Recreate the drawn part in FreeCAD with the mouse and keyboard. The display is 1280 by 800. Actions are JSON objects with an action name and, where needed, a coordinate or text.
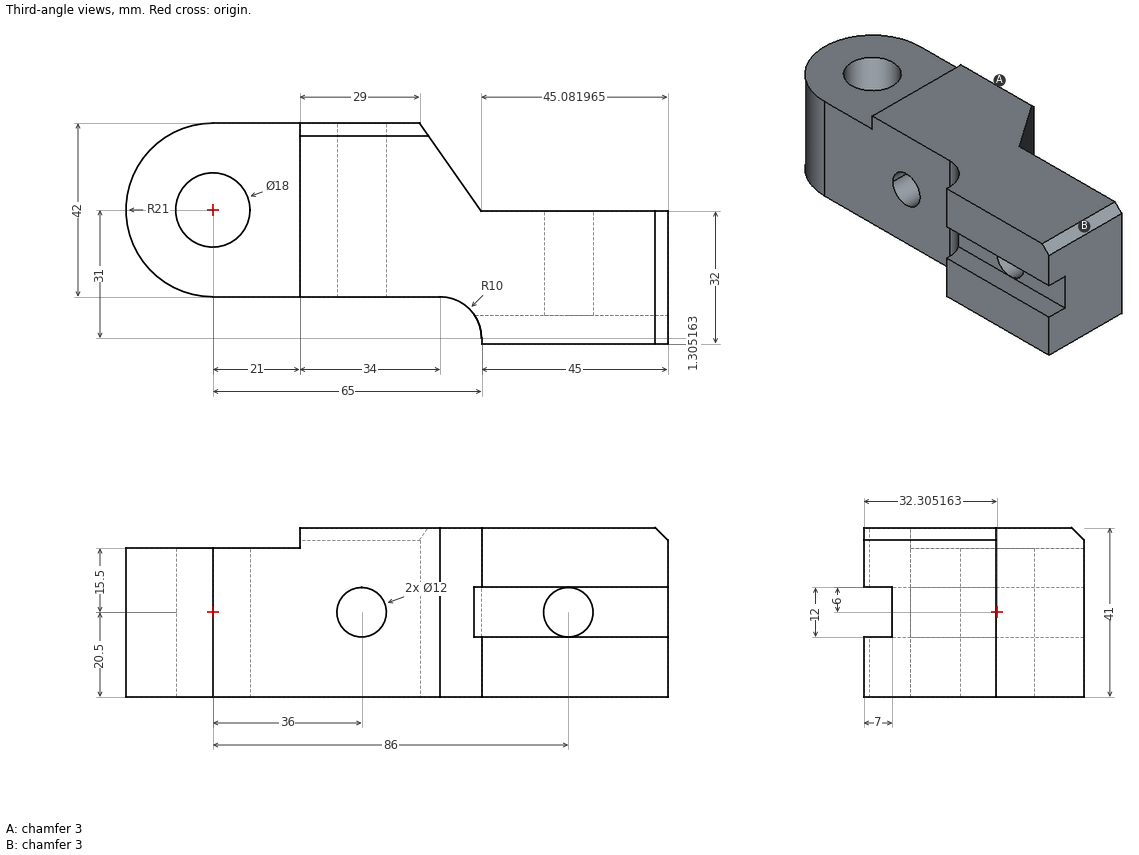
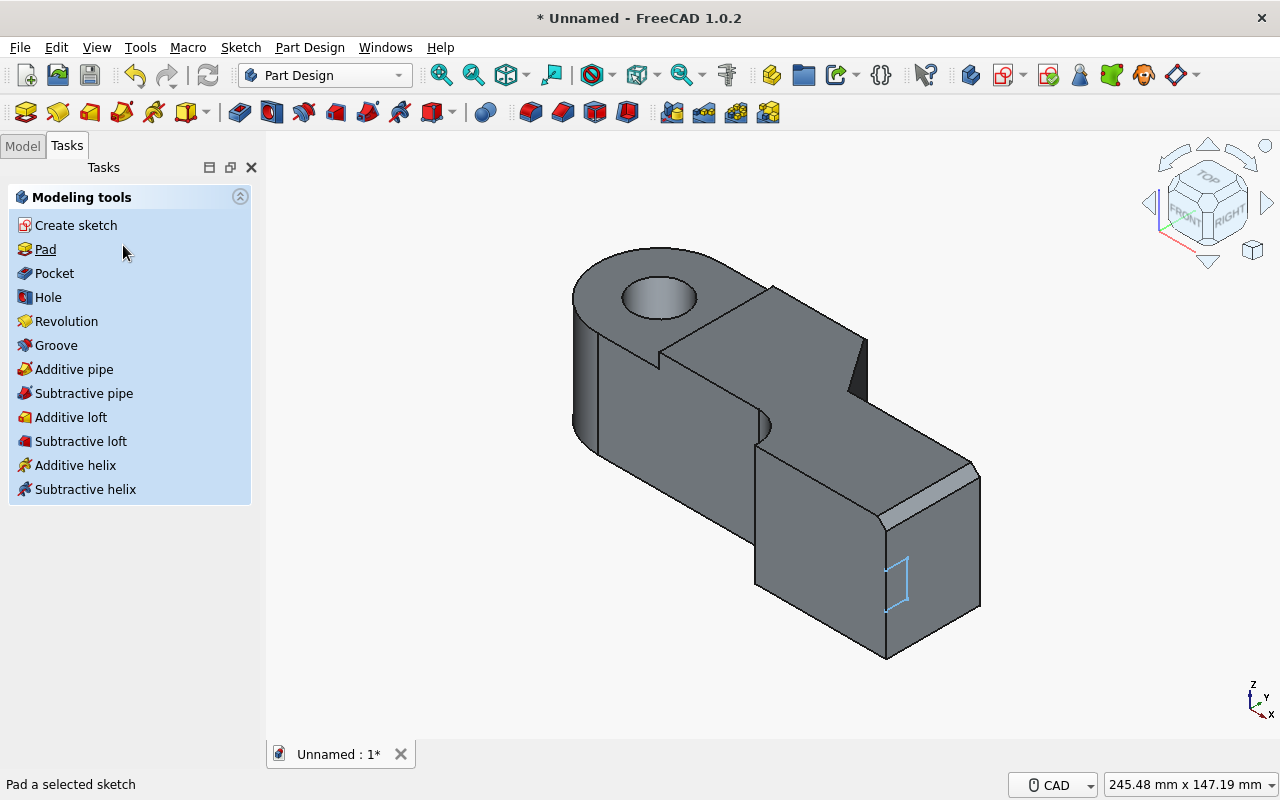
{"action": "left_click", "coordinate": [240, 112]}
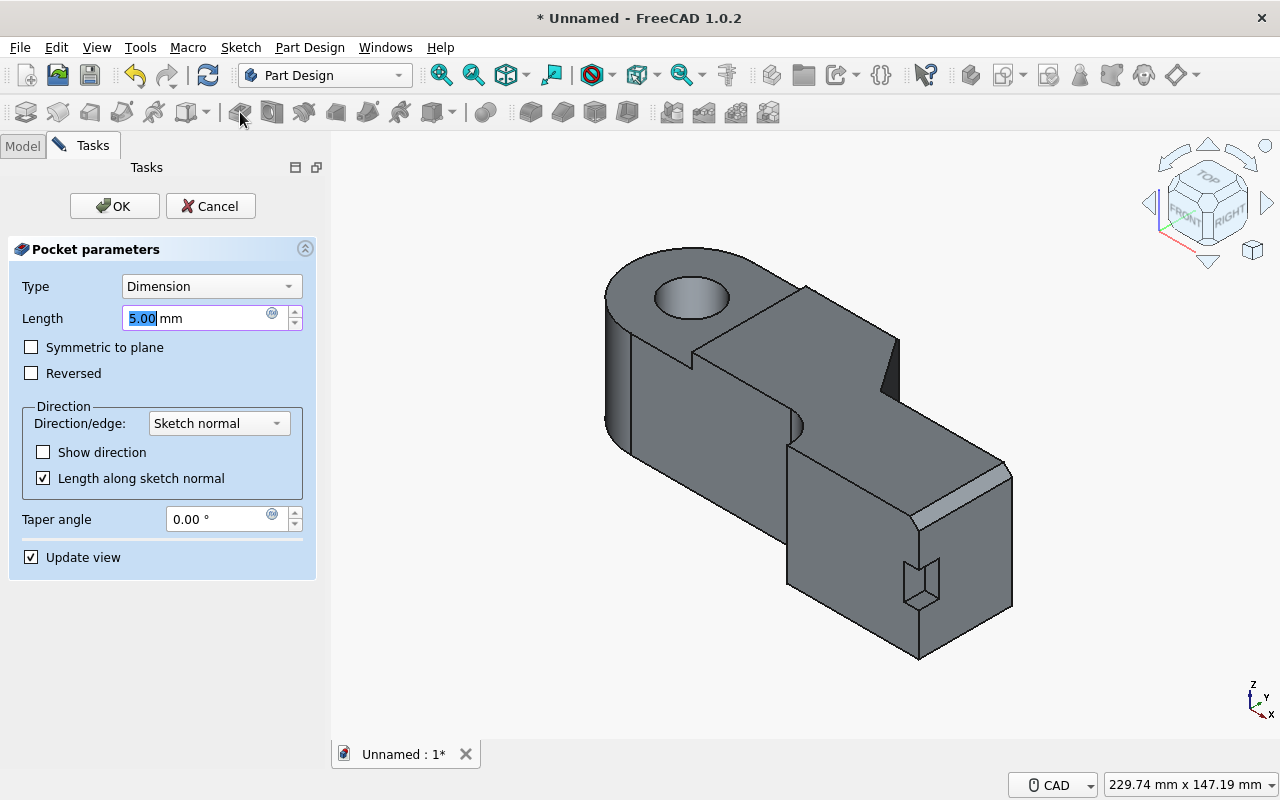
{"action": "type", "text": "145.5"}
{"action": "key", "text": "Tab"}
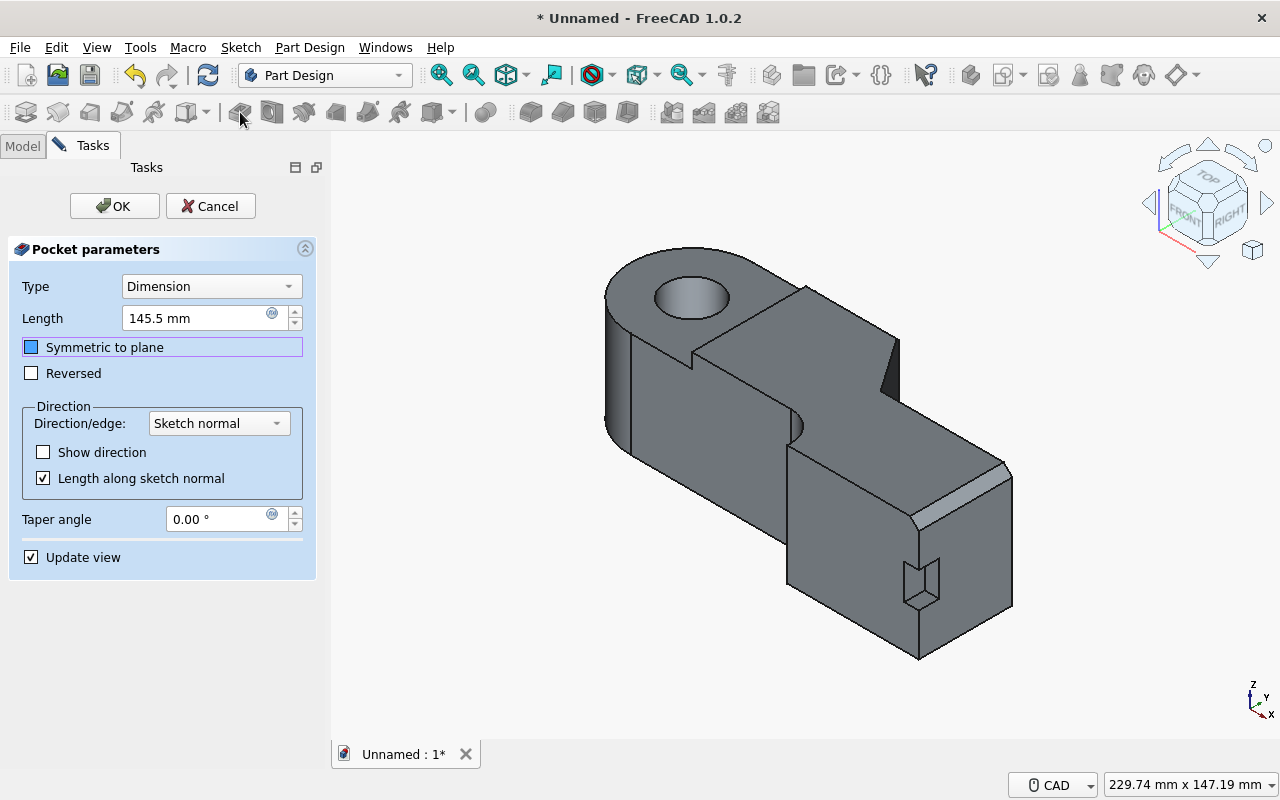
{"action": "left_click", "coordinate": [115, 206]}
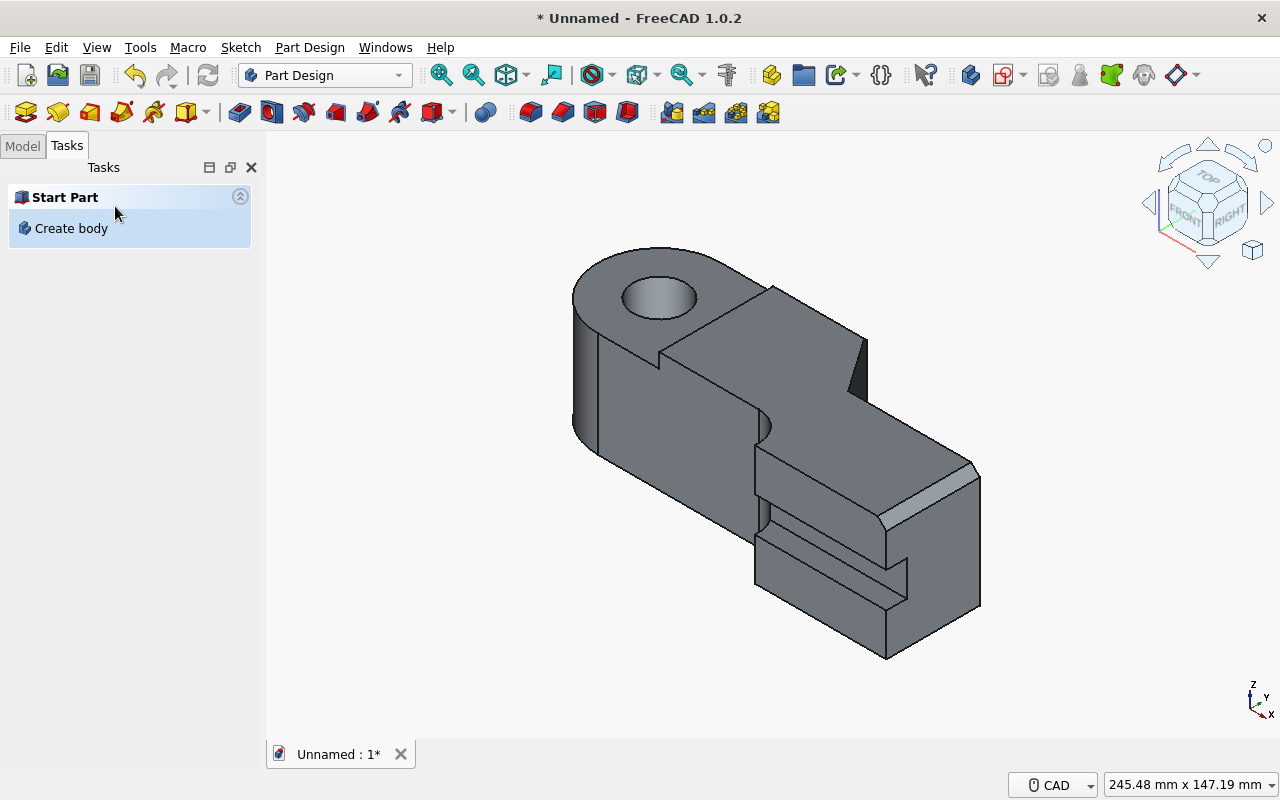
{"action": "key", "text": "4"}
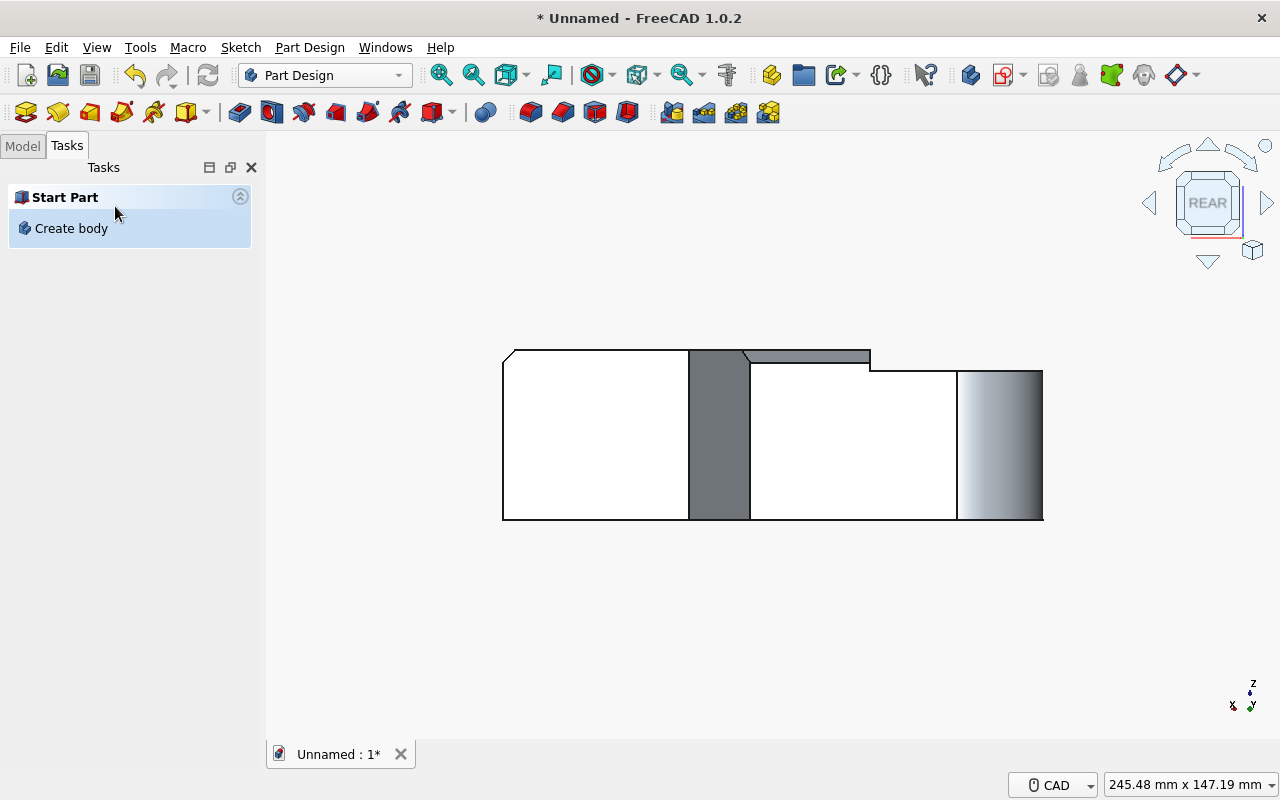
{"action": "left_click", "coordinate": [824, 440]}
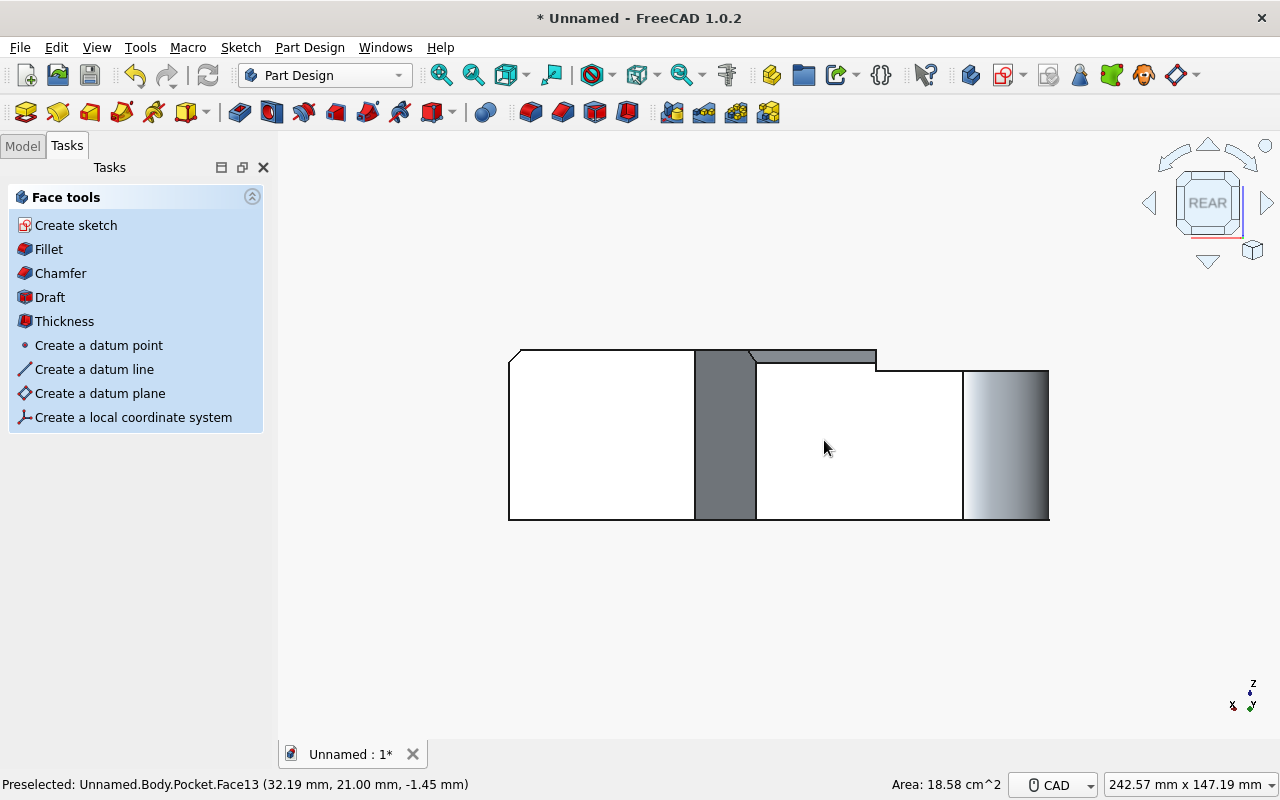
{"action": "left_click", "coordinate": [1004, 76]}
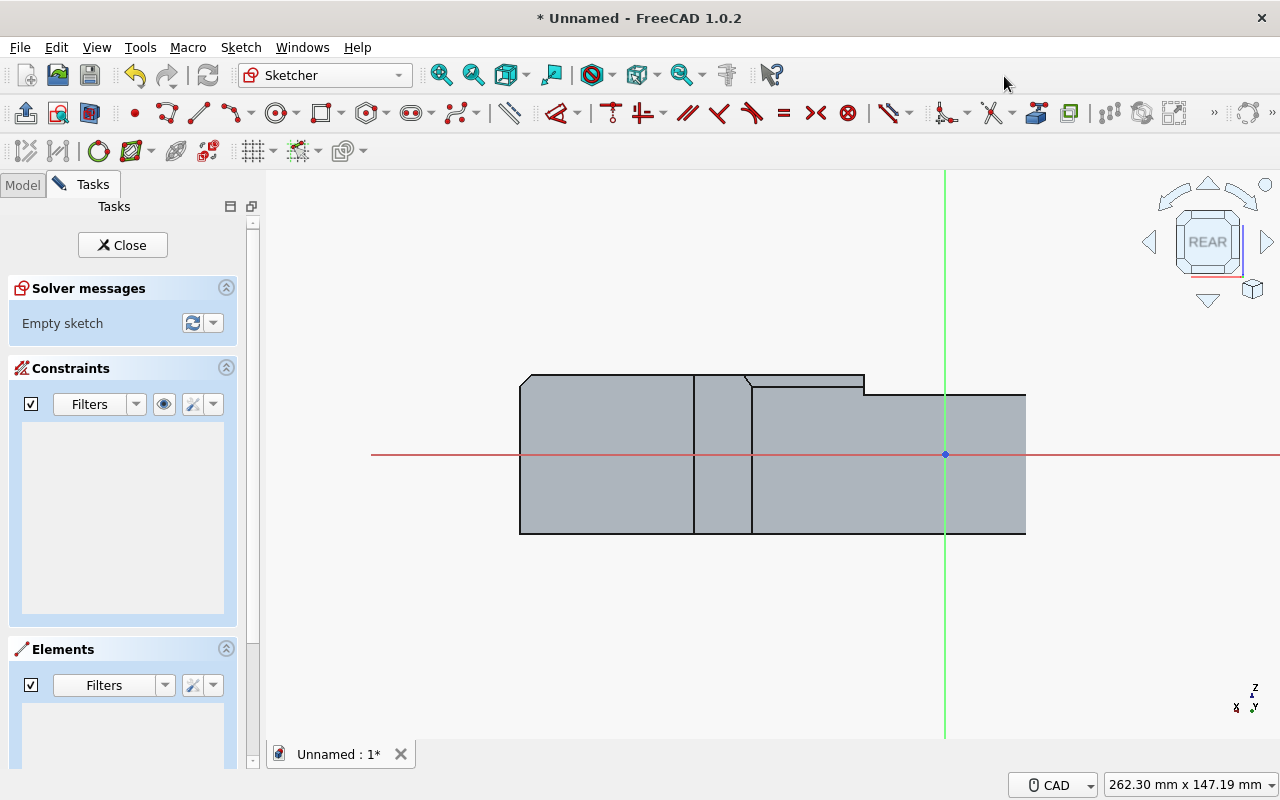
{"action": "scroll", "coordinate": [895, 455], "scroll_direction": "up", "scroll_amount": 2}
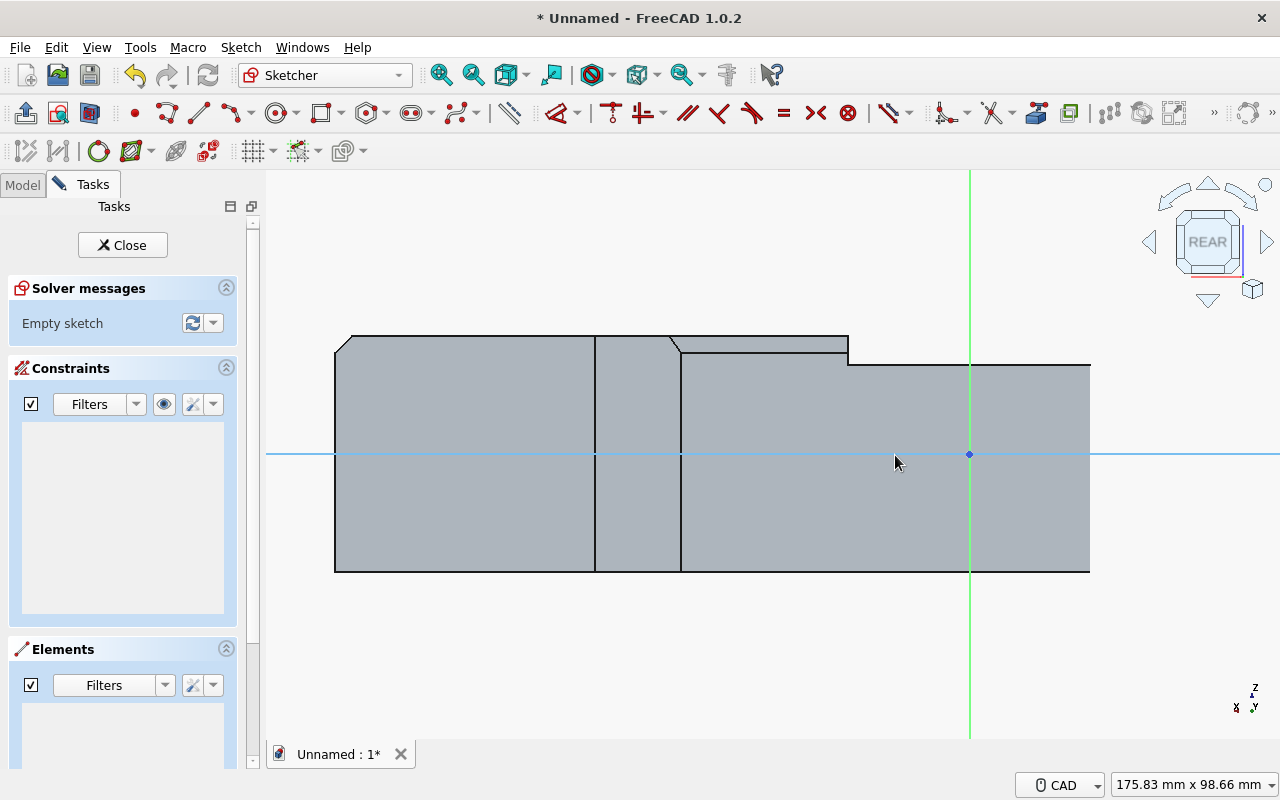
{"action": "left_click", "coordinate": [276, 114]}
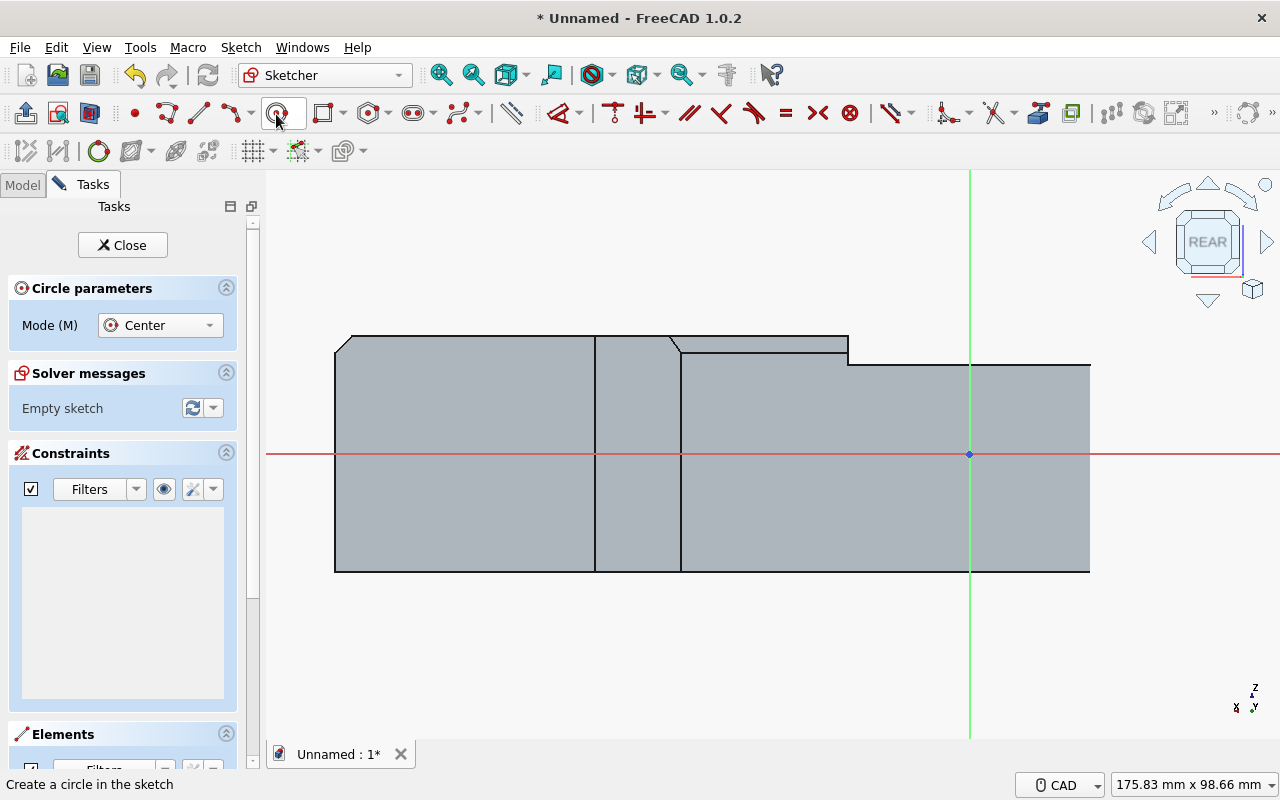
{"action": "left_click", "coordinate": [762, 454]}
{"action": "mouse_move", "coordinate": [786, 430]}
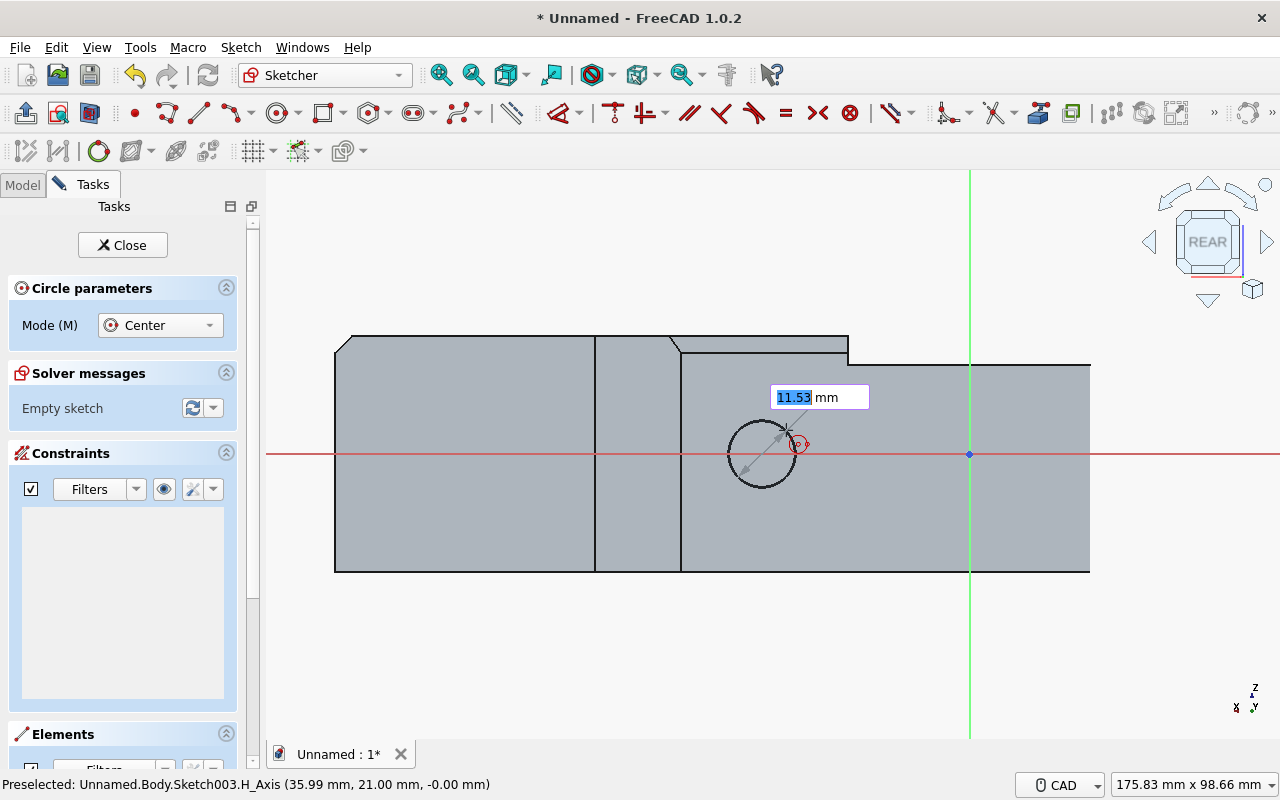
{"action": "type", "text": "12"}
{"action": "key", "text": "Return"}